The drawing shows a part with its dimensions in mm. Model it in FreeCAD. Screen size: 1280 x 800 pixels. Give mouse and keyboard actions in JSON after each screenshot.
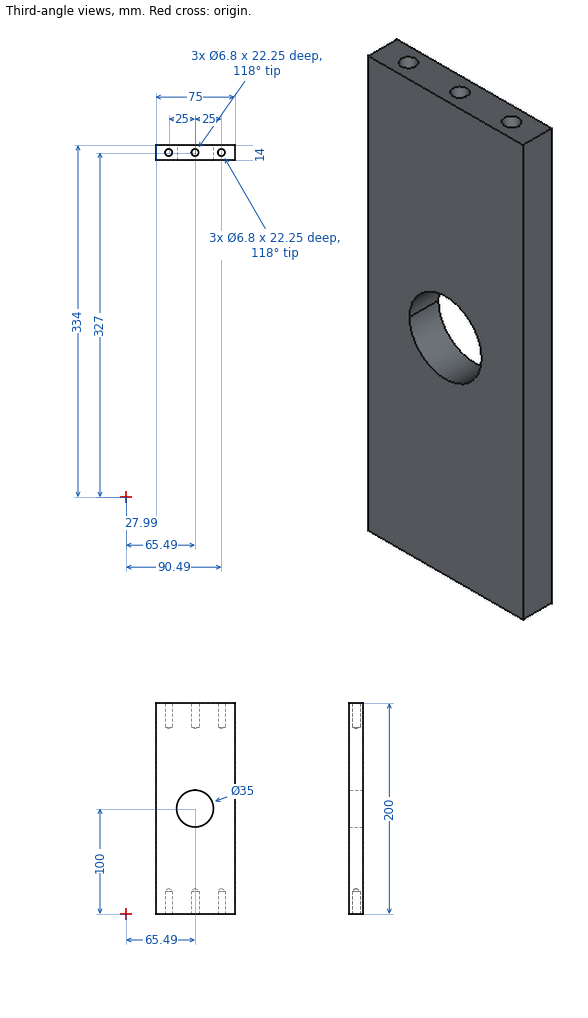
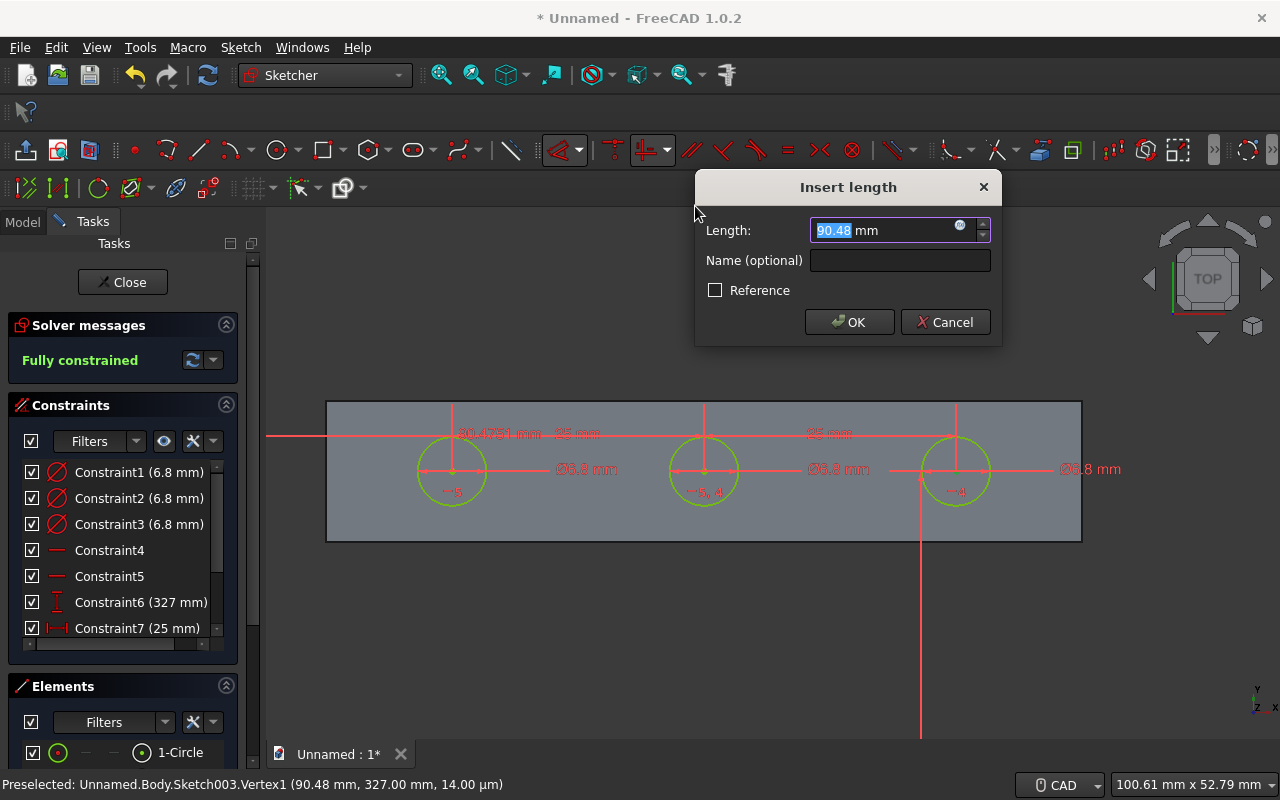
{"action": "type", "text": "90.49"}
{"action": "key", "text": "Return"}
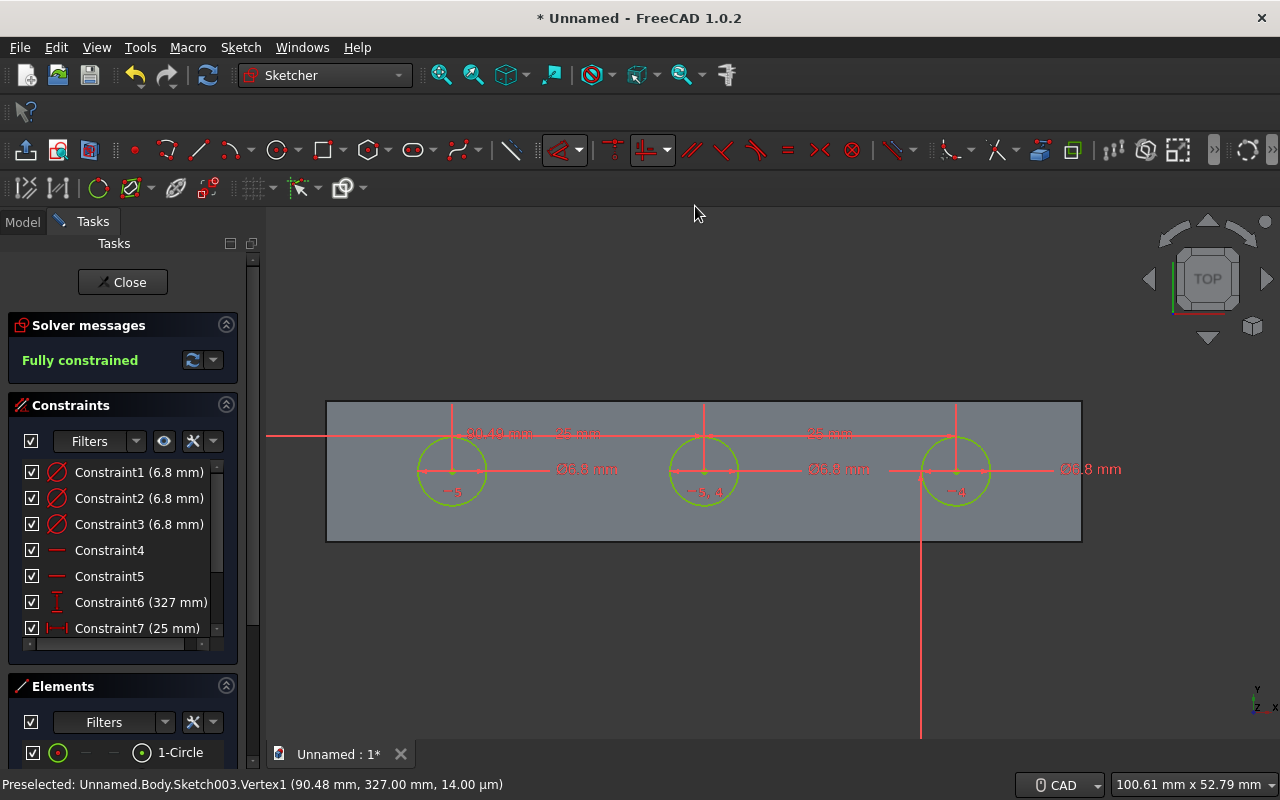
{"action": "left_click", "coordinate": [123, 282]}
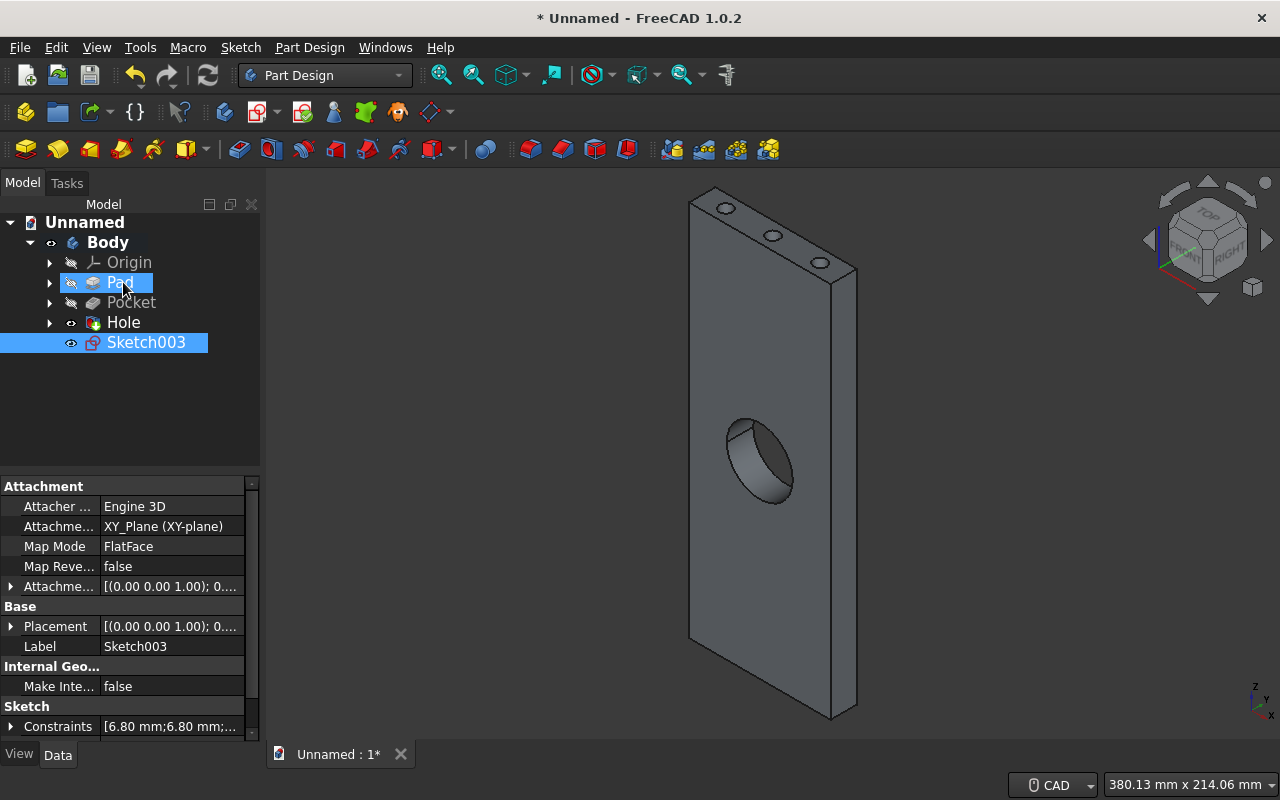
{"action": "left_click", "coordinate": [272, 150]}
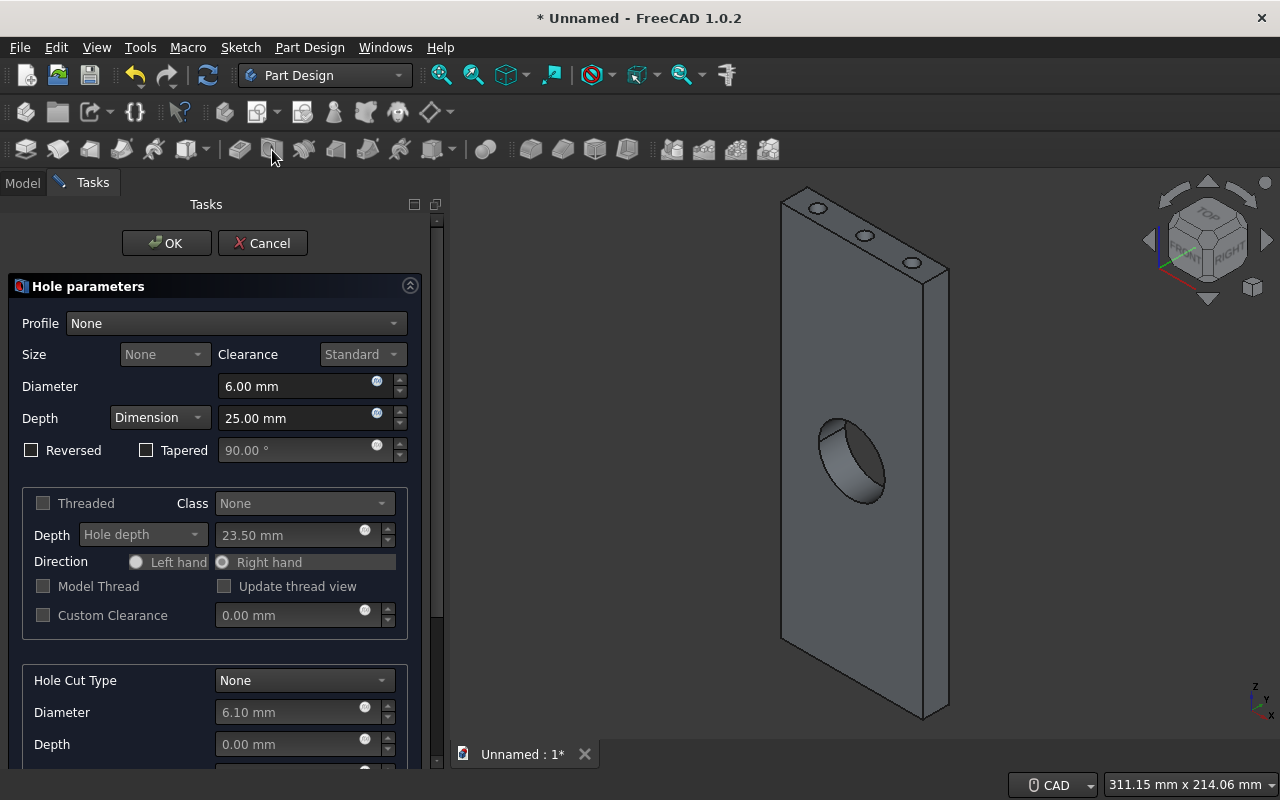
{"action": "triple_click", "coordinate": [305, 386]}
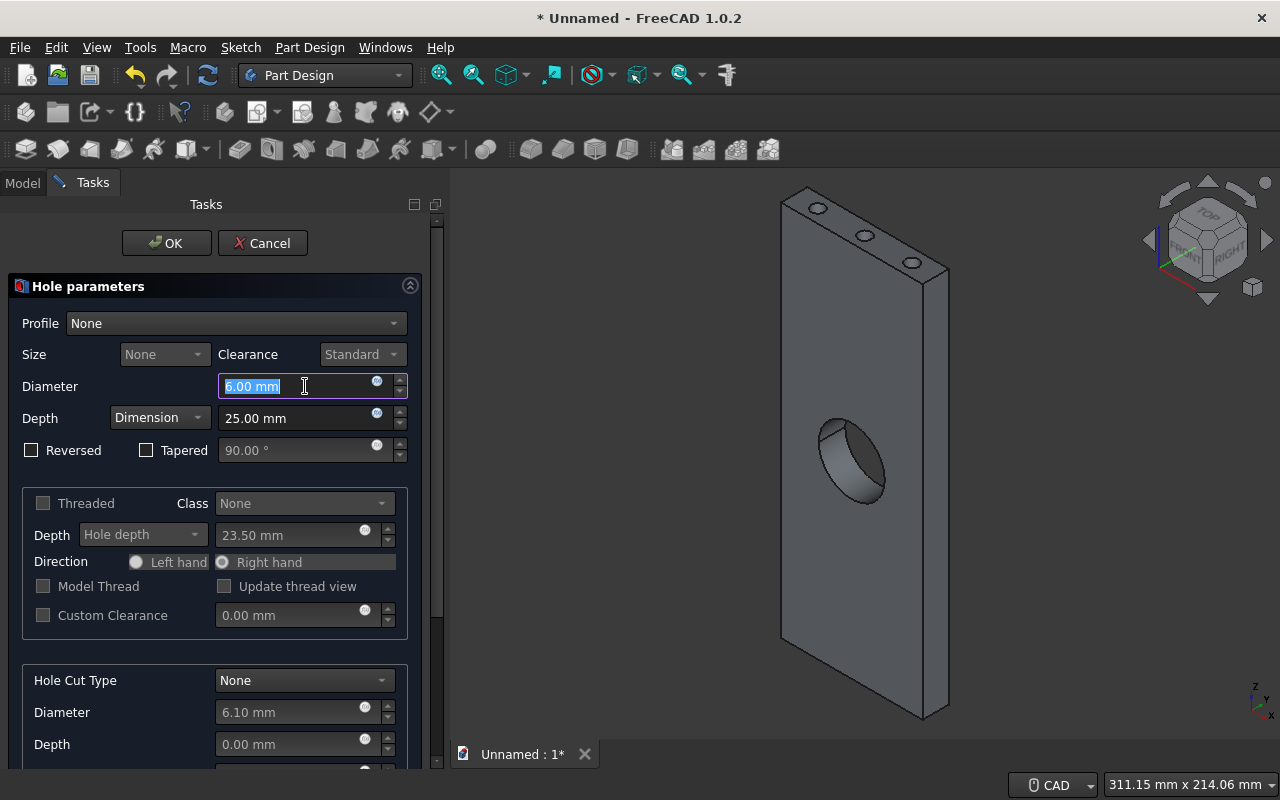
{"action": "type", "text": "6.8"}
{"action": "key", "text": "Tab"}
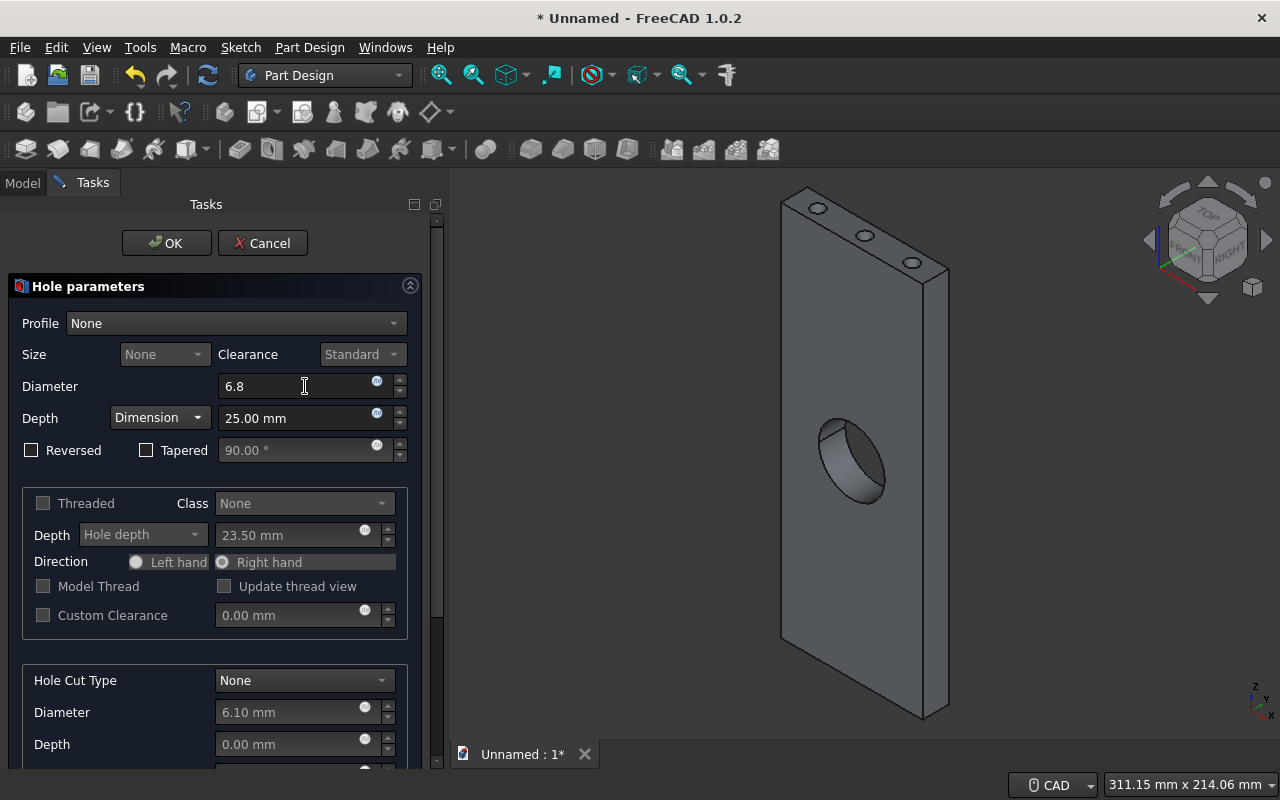
{"action": "triple_click", "coordinate": [305, 418]}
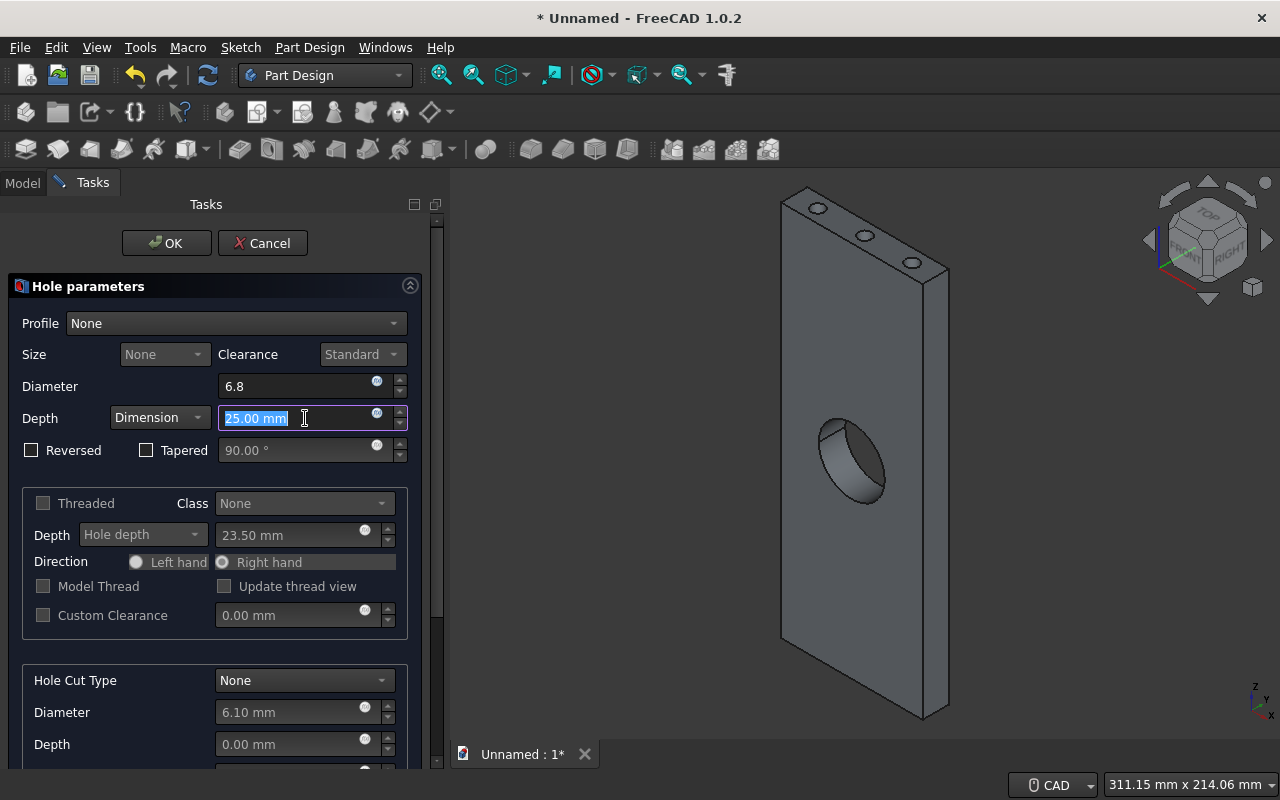
{"action": "type", "text": "22.25"}
{"action": "key", "text": "Tab"}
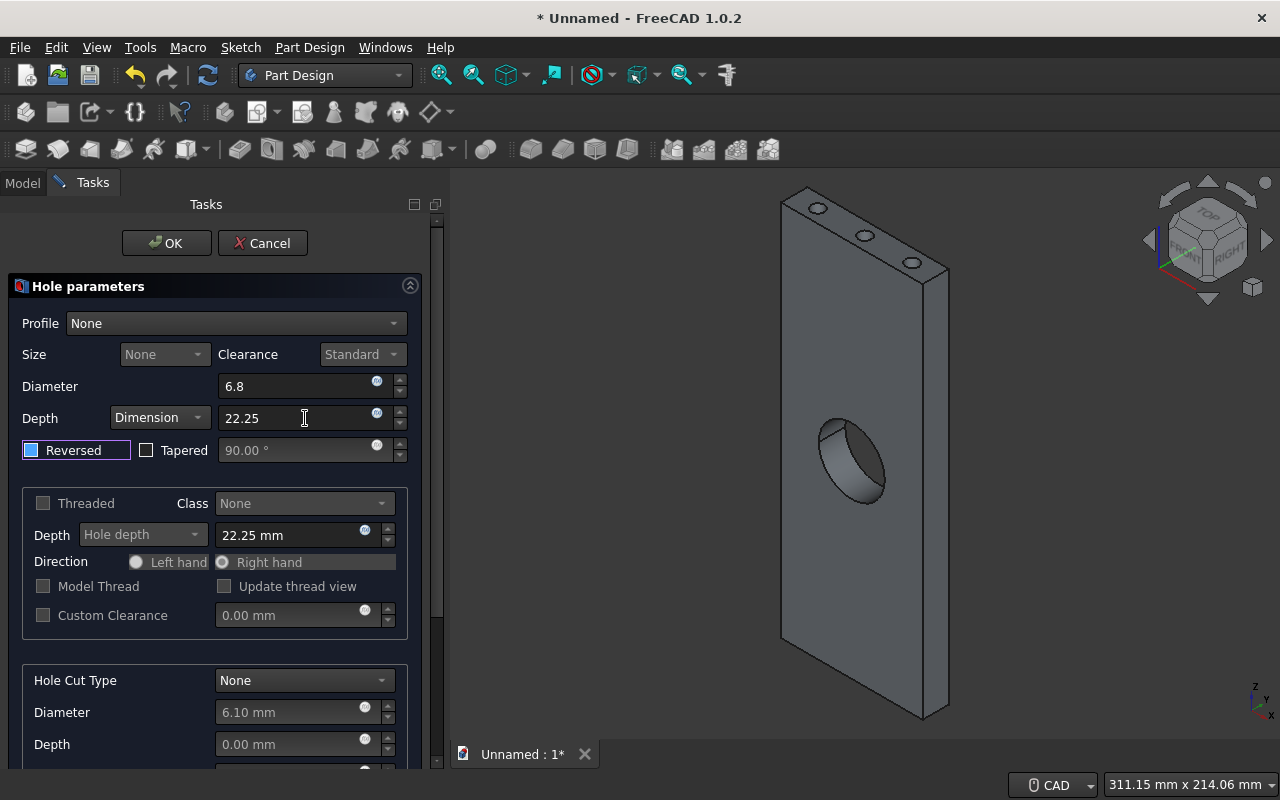
{"action": "left_click", "coordinate": [30, 450]}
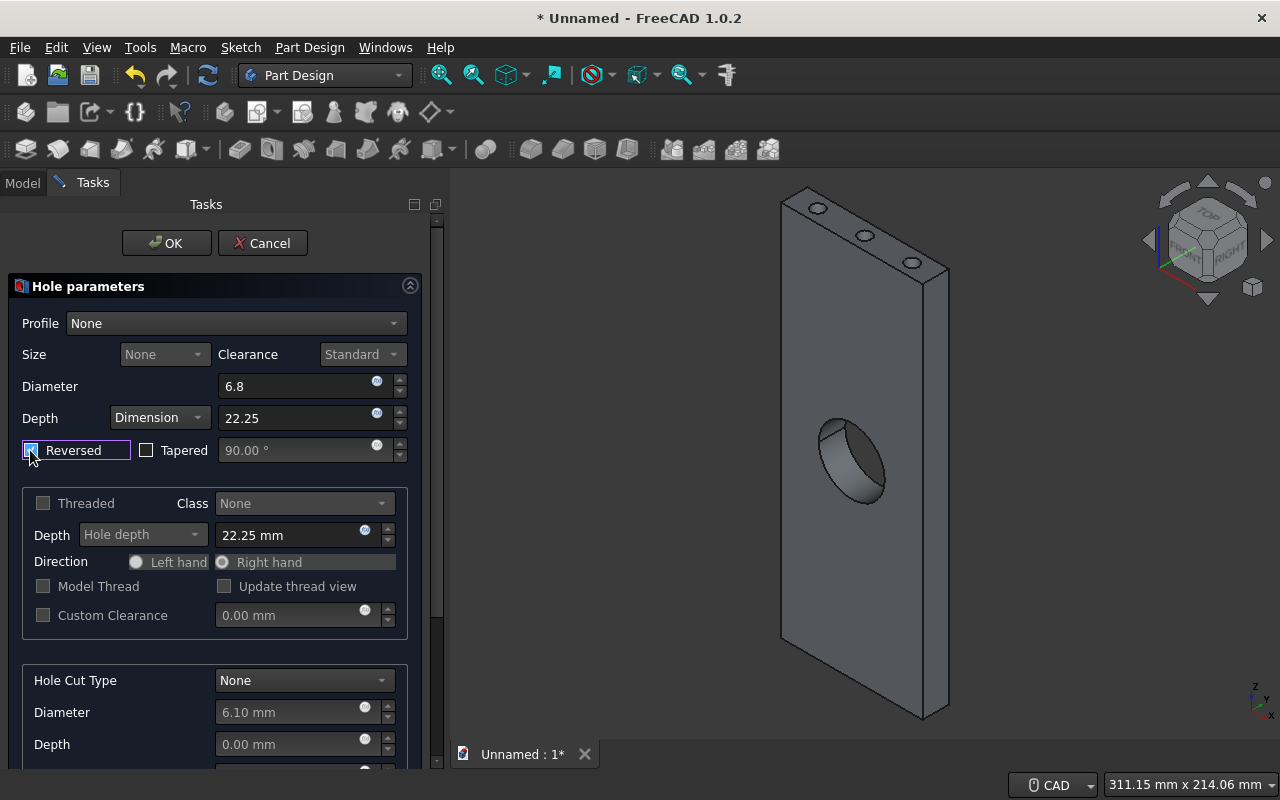
{"action": "left_click", "coordinate": [167, 243]}